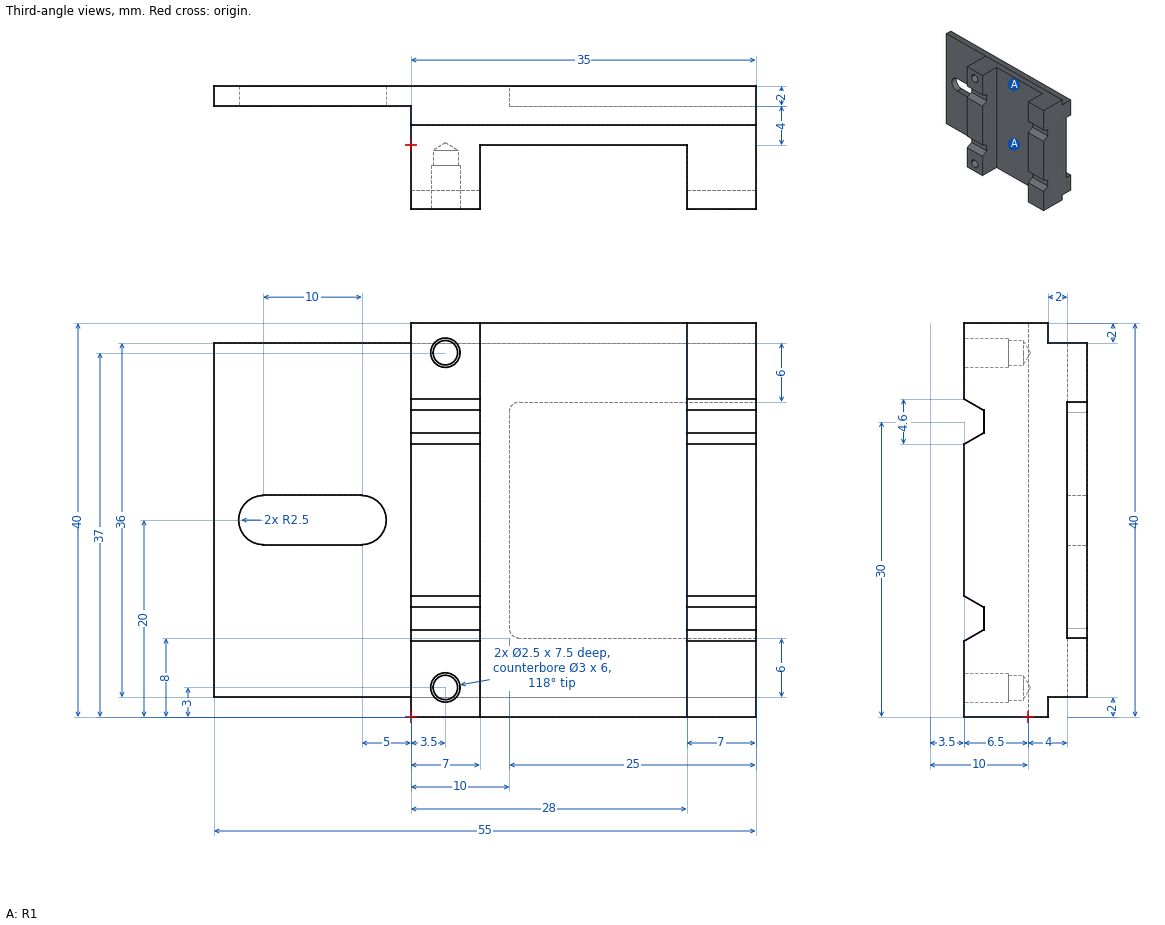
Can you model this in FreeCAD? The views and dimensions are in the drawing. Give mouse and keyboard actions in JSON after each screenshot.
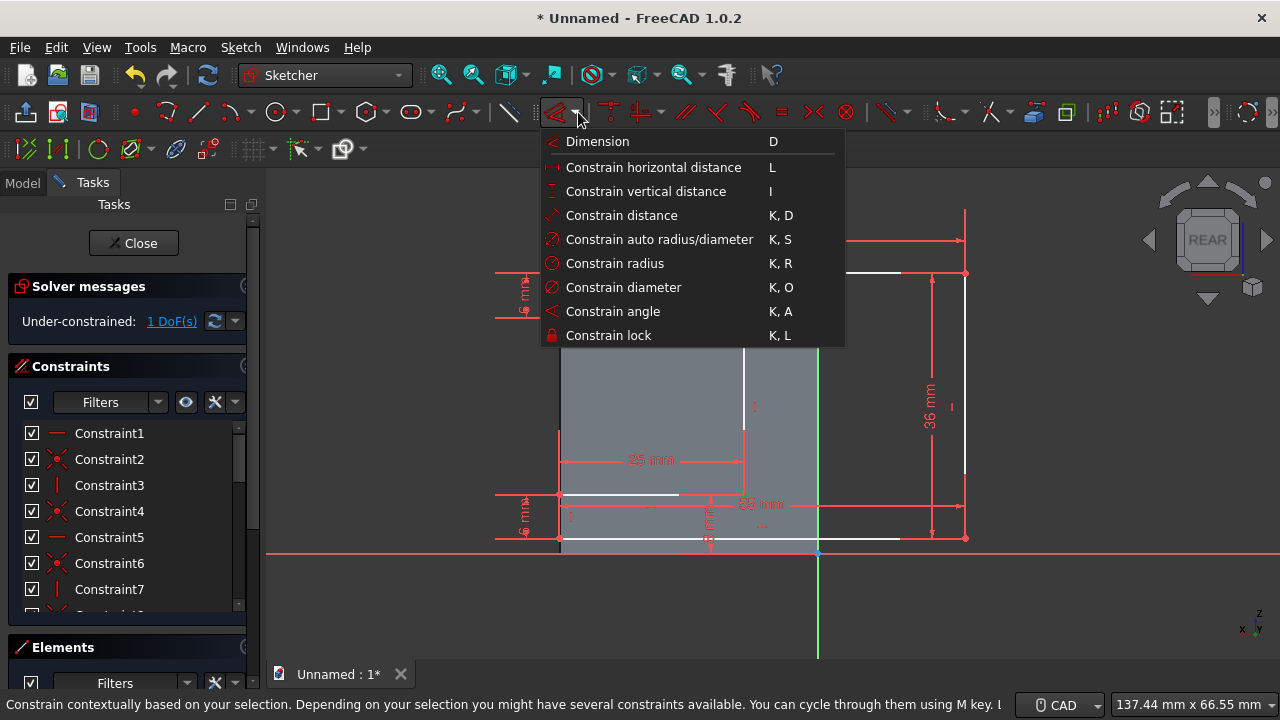
{"action": "left_click", "coordinate": [693, 167]}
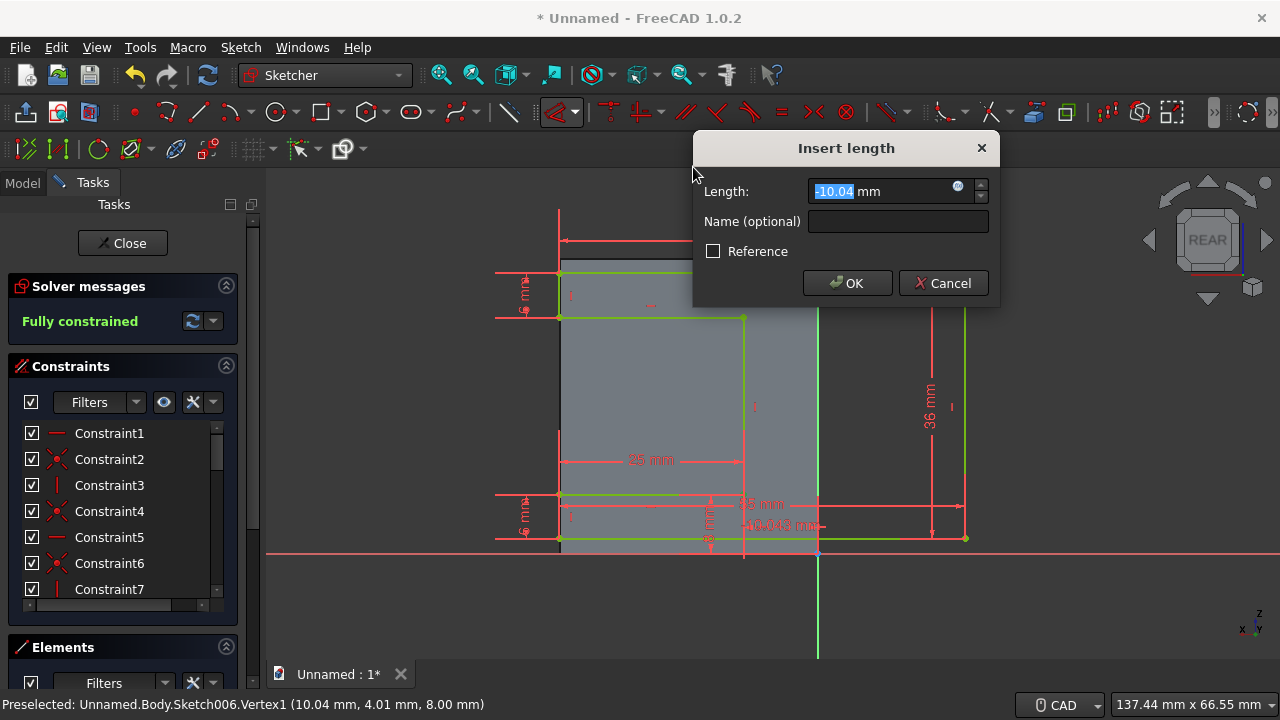
{"action": "type", "text": "-10"}
{"action": "key", "text": "Return"}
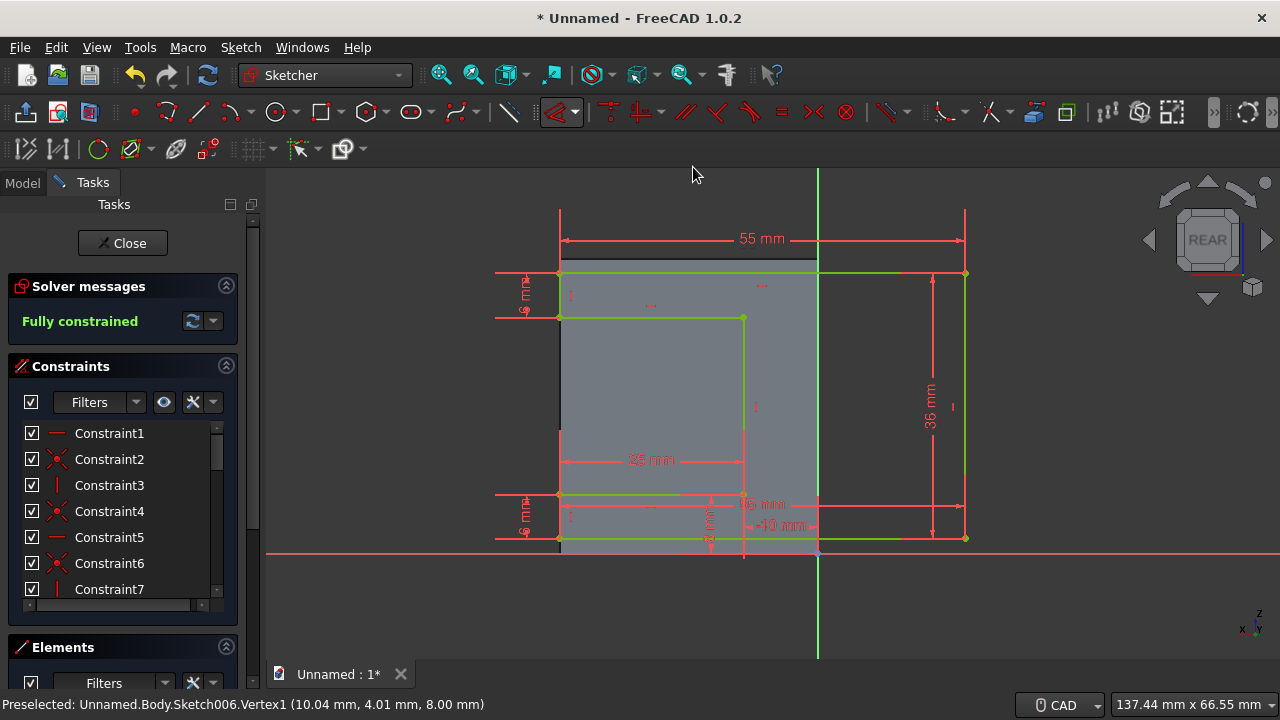
{"action": "left_click", "coordinate": [123, 243]}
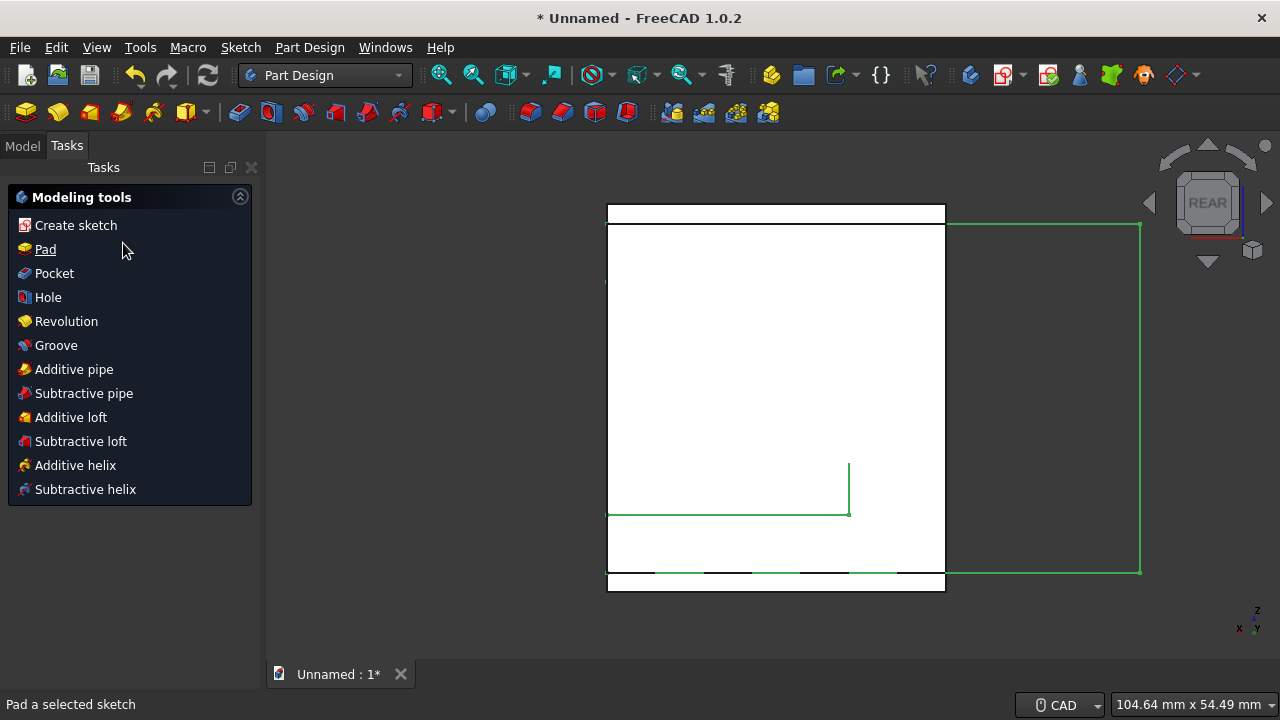
{"action": "left_click", "coordinate": [26, 112]}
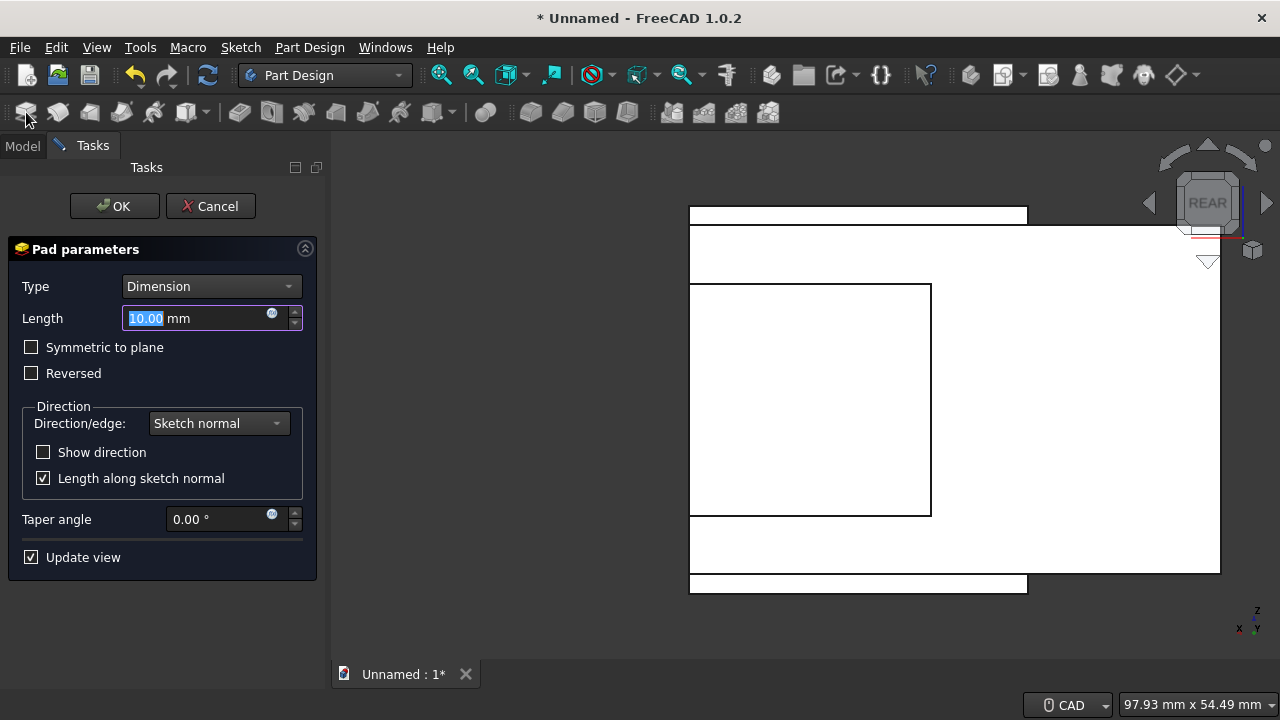
{"action": "type", "text": "2"}
{"action": "key", "text": "Tab"}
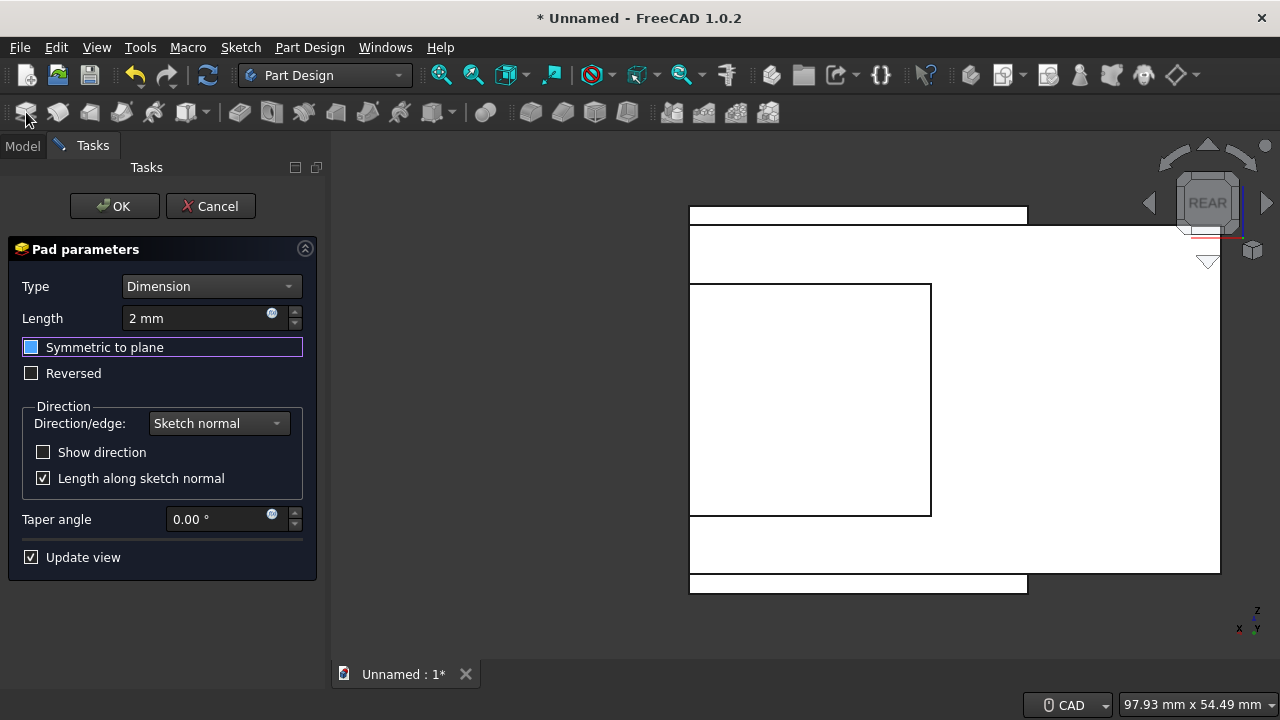
{"action": "left_click", "coordinate": [115, 206]}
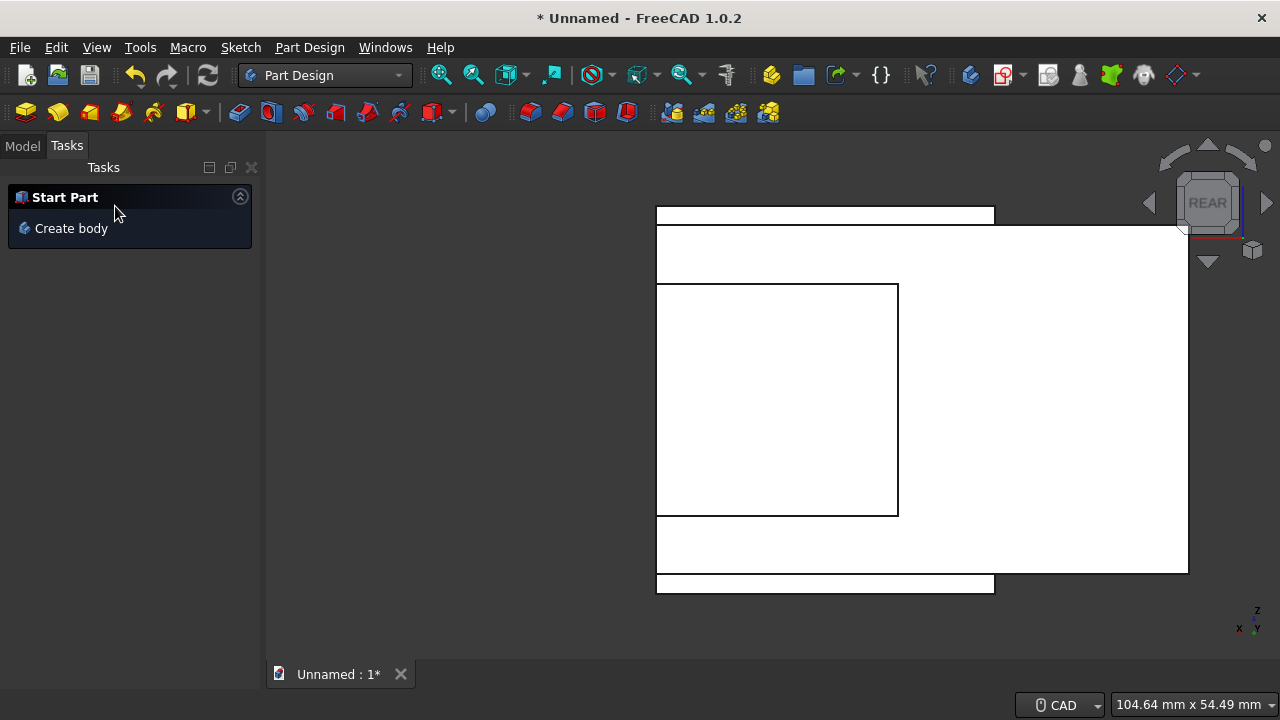
{"action": "key", "text": "6"}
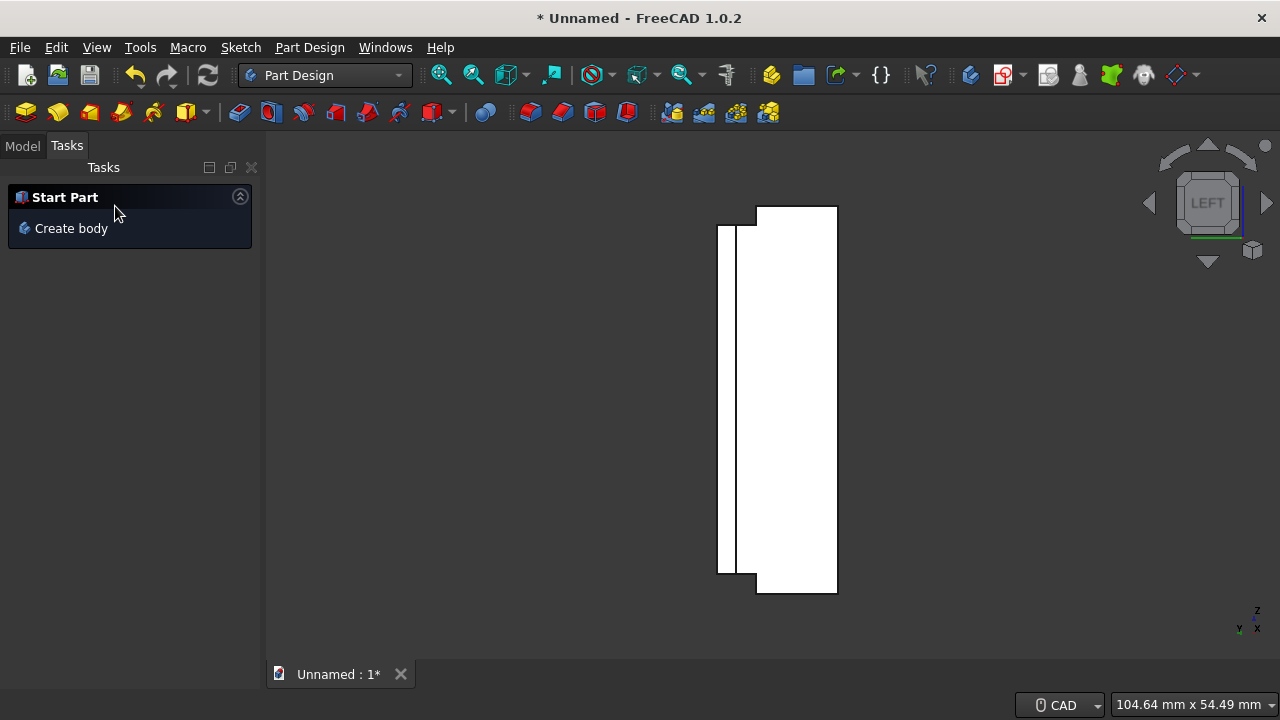
{"action": "left_click", "coordinate": [787, 288]}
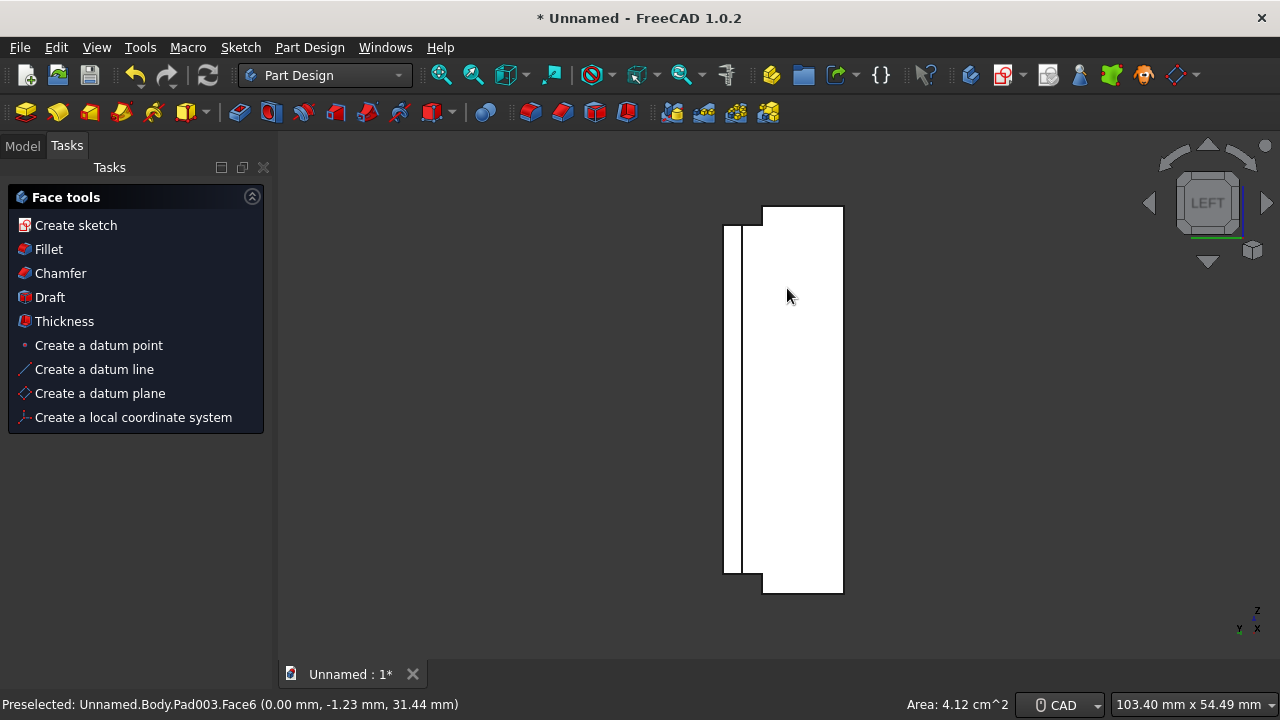
{"action": "left_click", "coordinate": [1004, 76]}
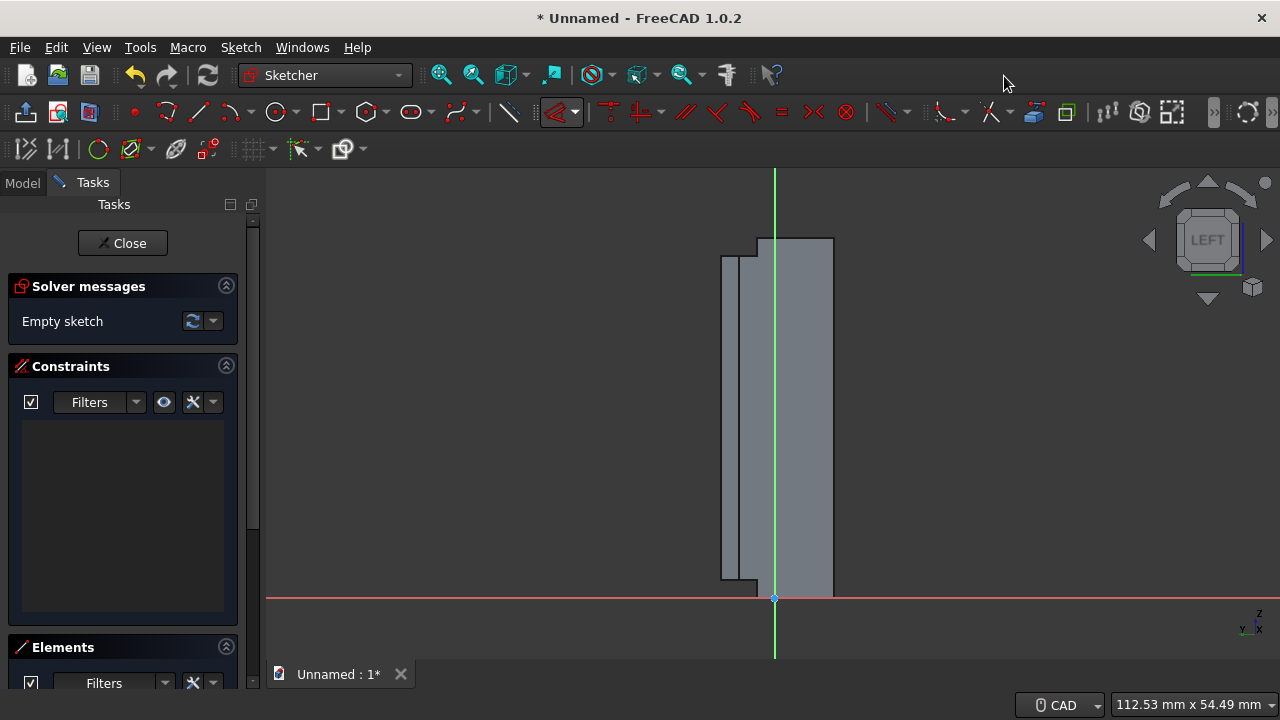
{"action": "scroll", "coordinate": [854, 315], "scroll_direction": "up", "scroll_amount": 10}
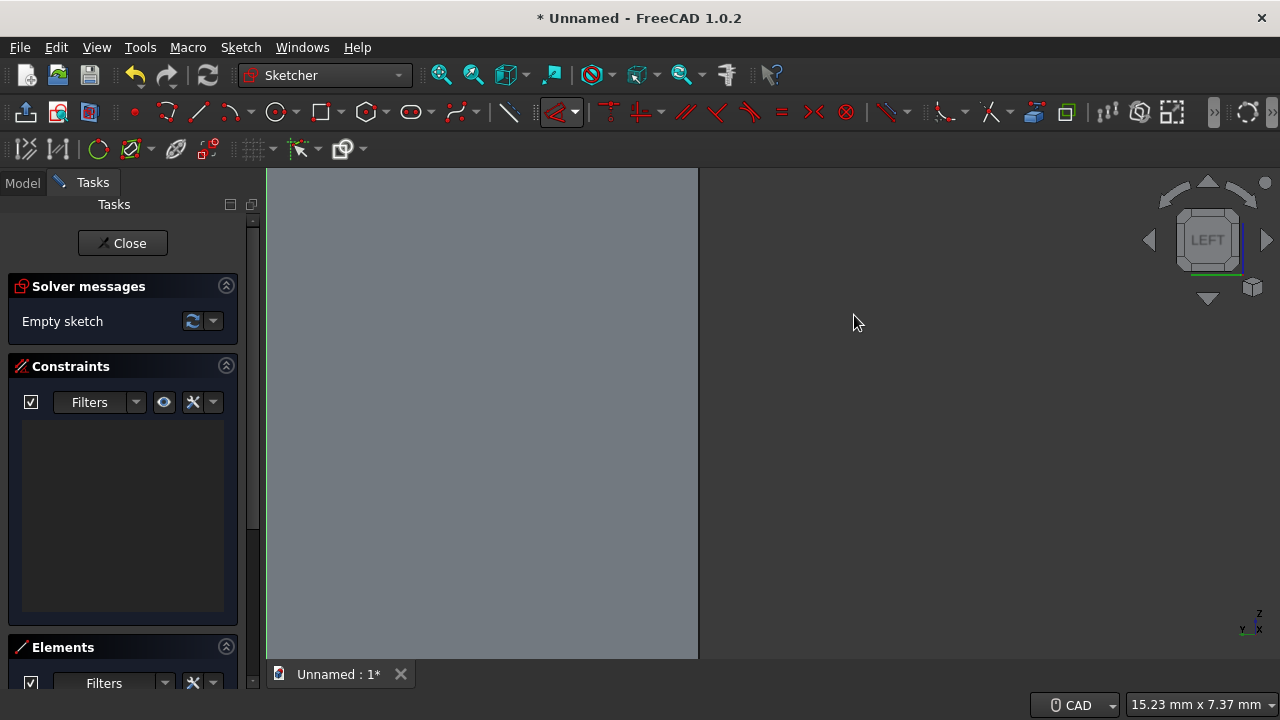
{"action": "left_click", "coordinate": [366, 112]}